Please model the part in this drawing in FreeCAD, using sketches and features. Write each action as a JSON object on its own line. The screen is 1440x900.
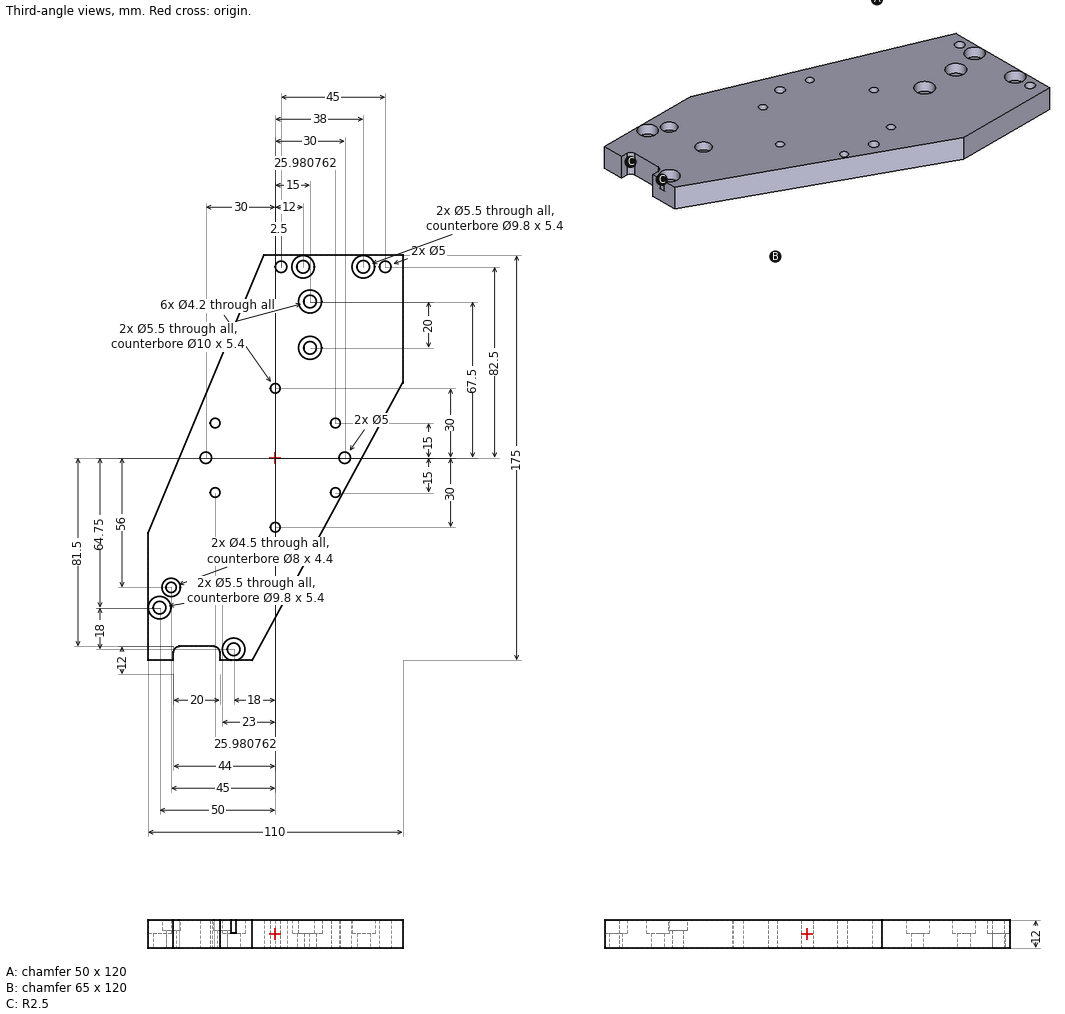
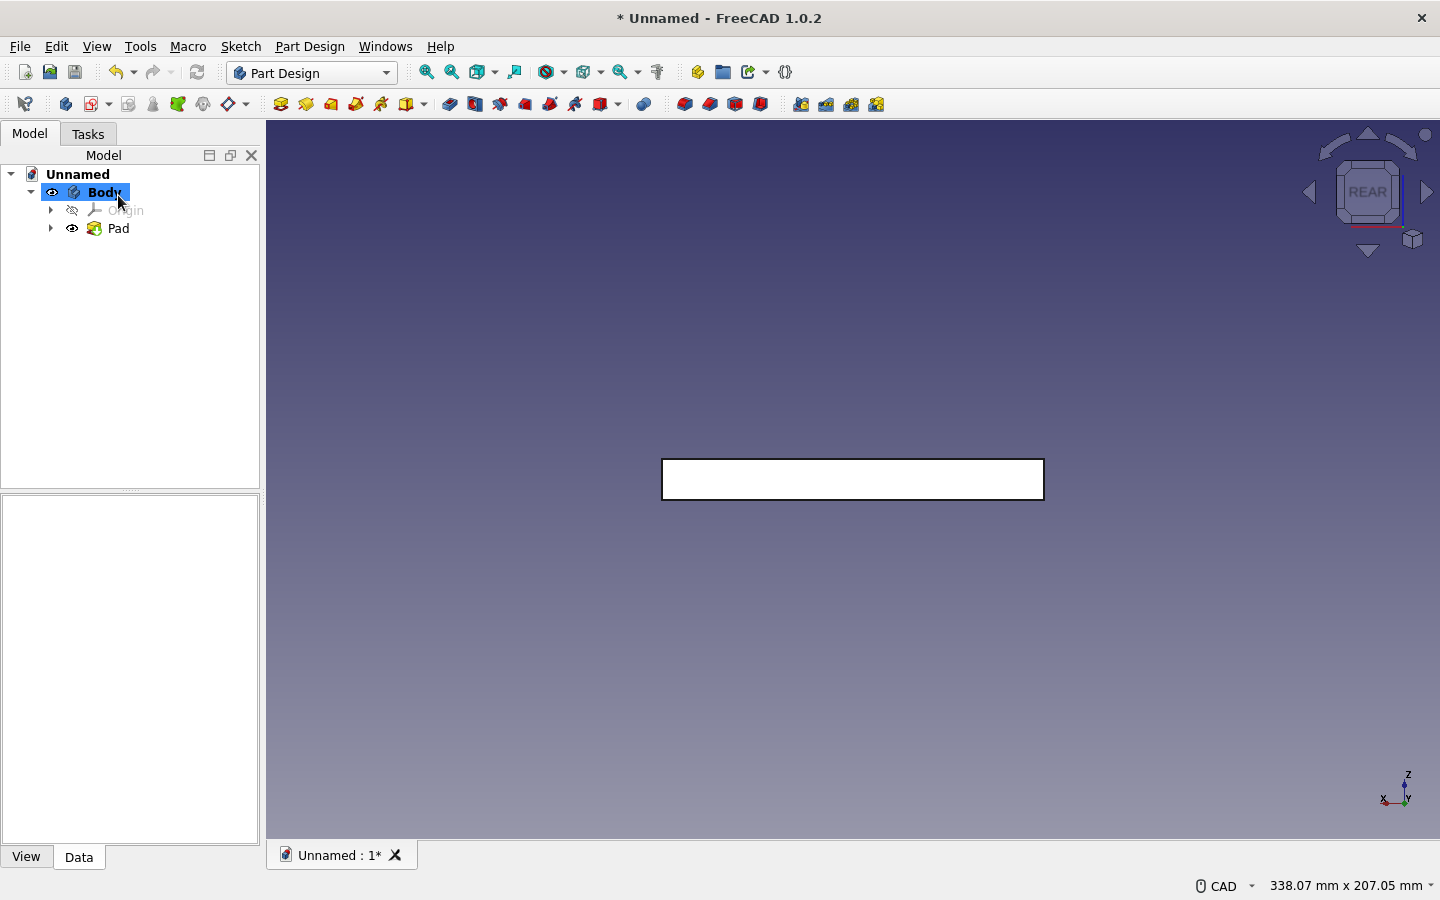
{"action": "left_click", "coordinate": [1044, 479]}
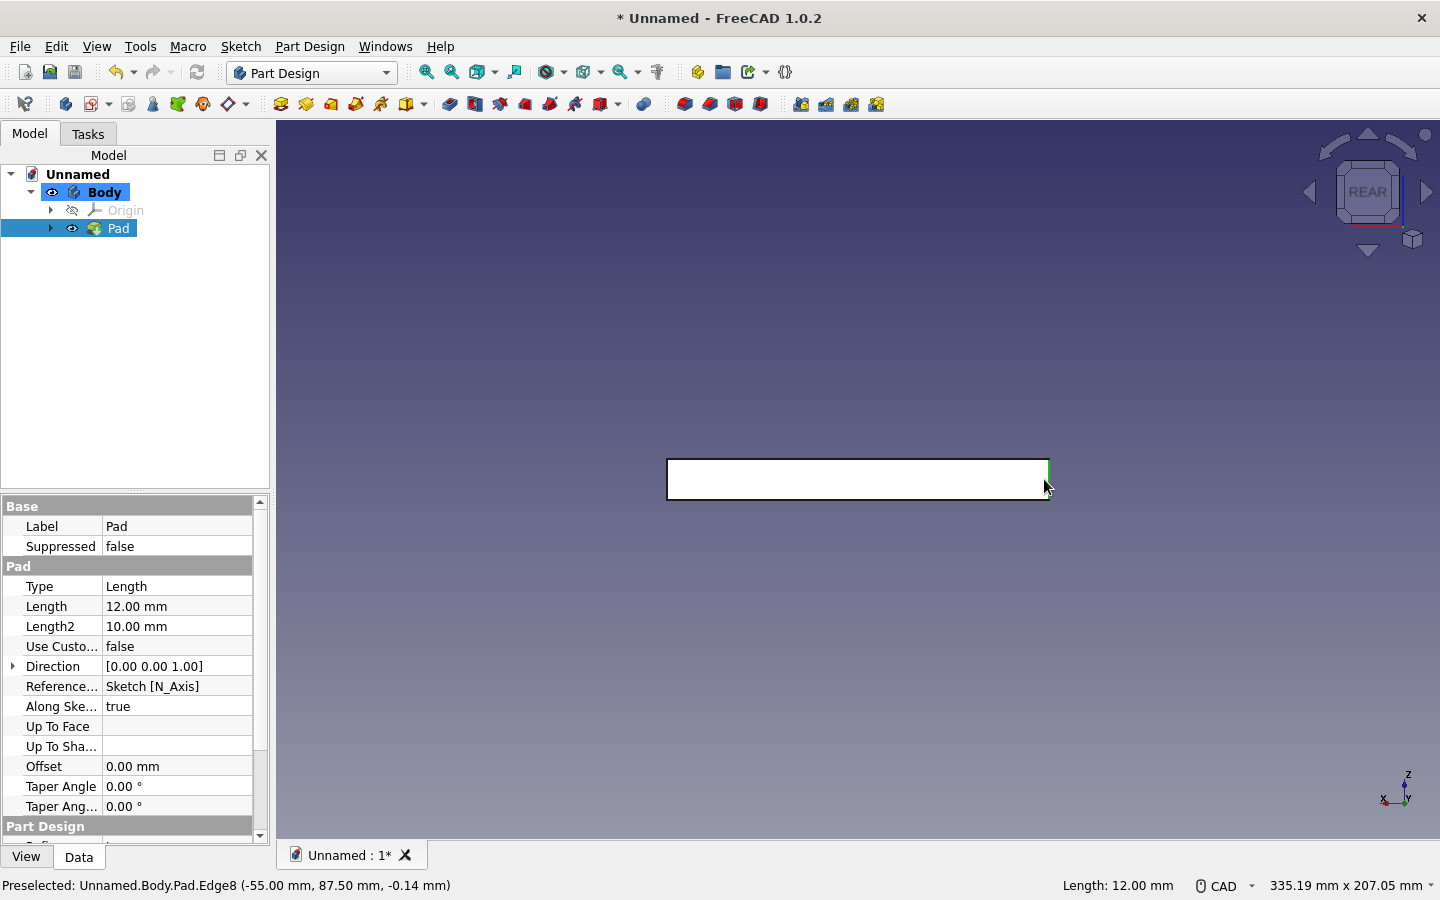
{"action": "left_click", "coordinate": [710, 104]}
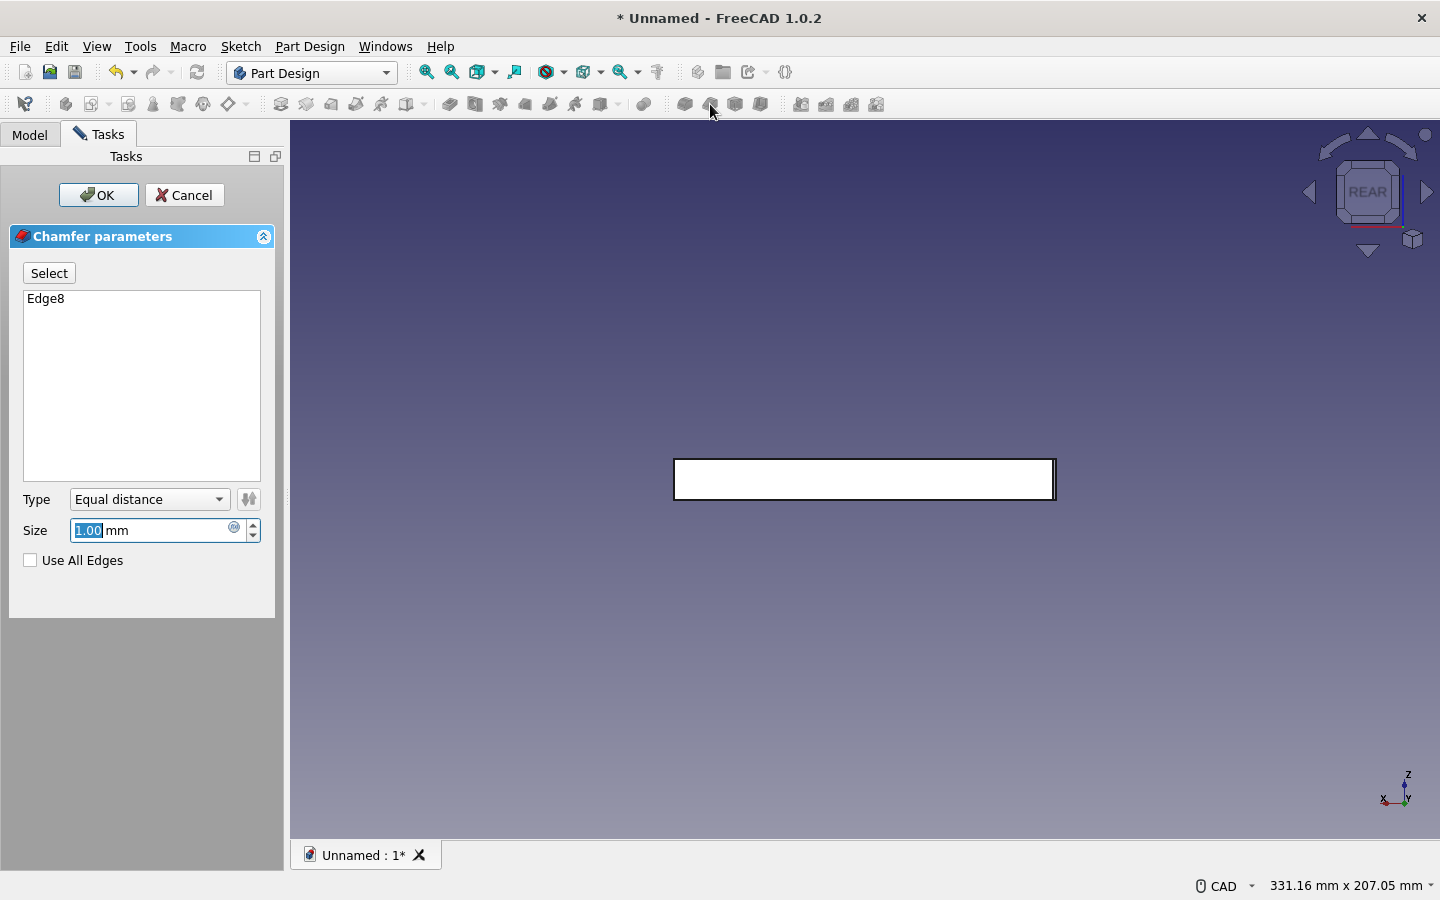
{"action": "type", "text": "50"}
{"action": "key", "text": "Tab"}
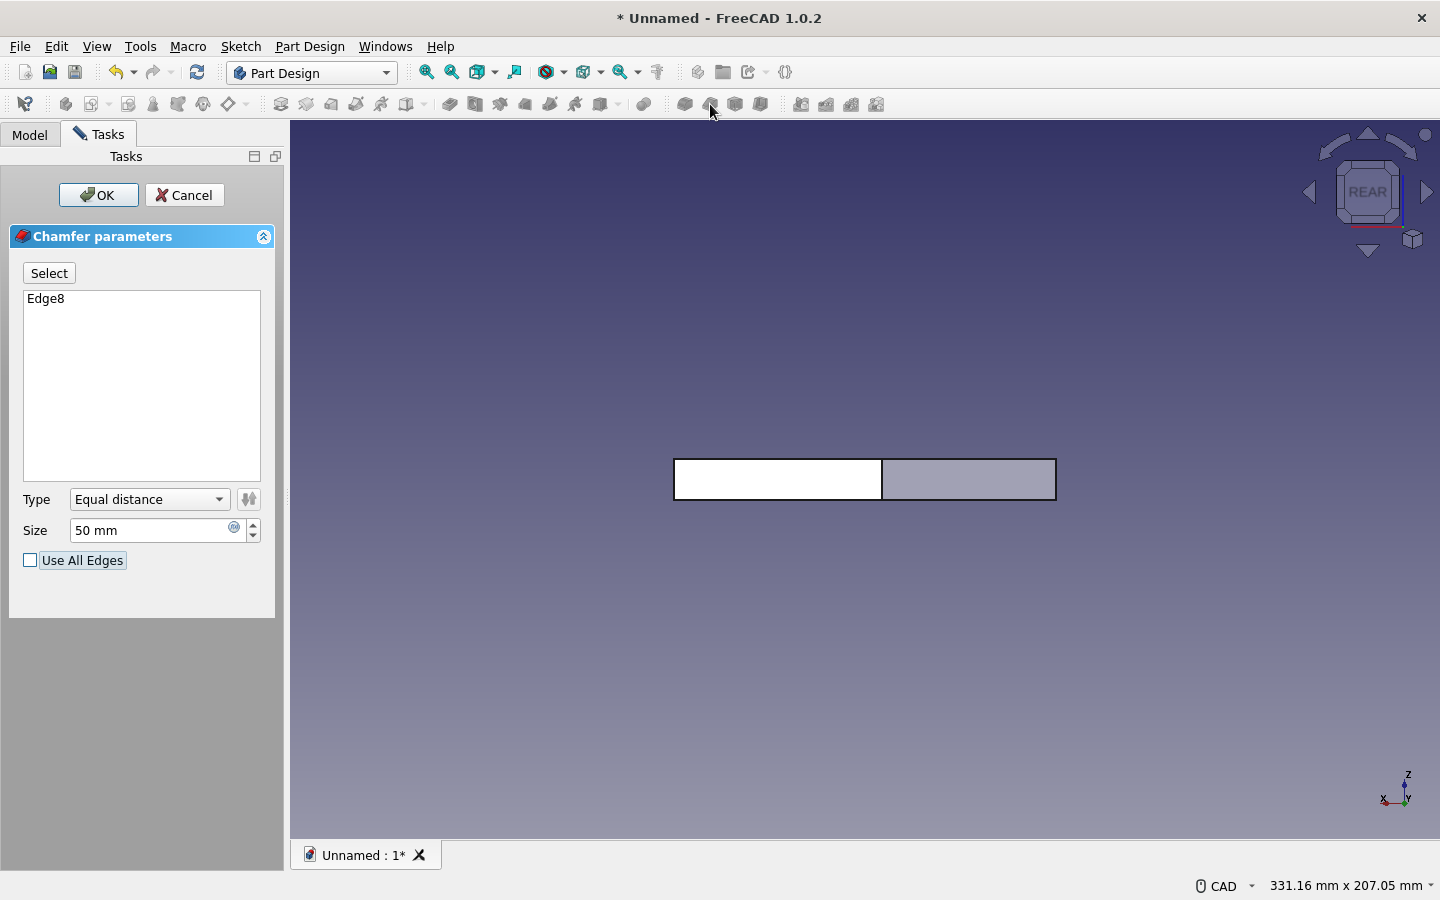
{"action": "left_click", "coordinate": [150, 500]}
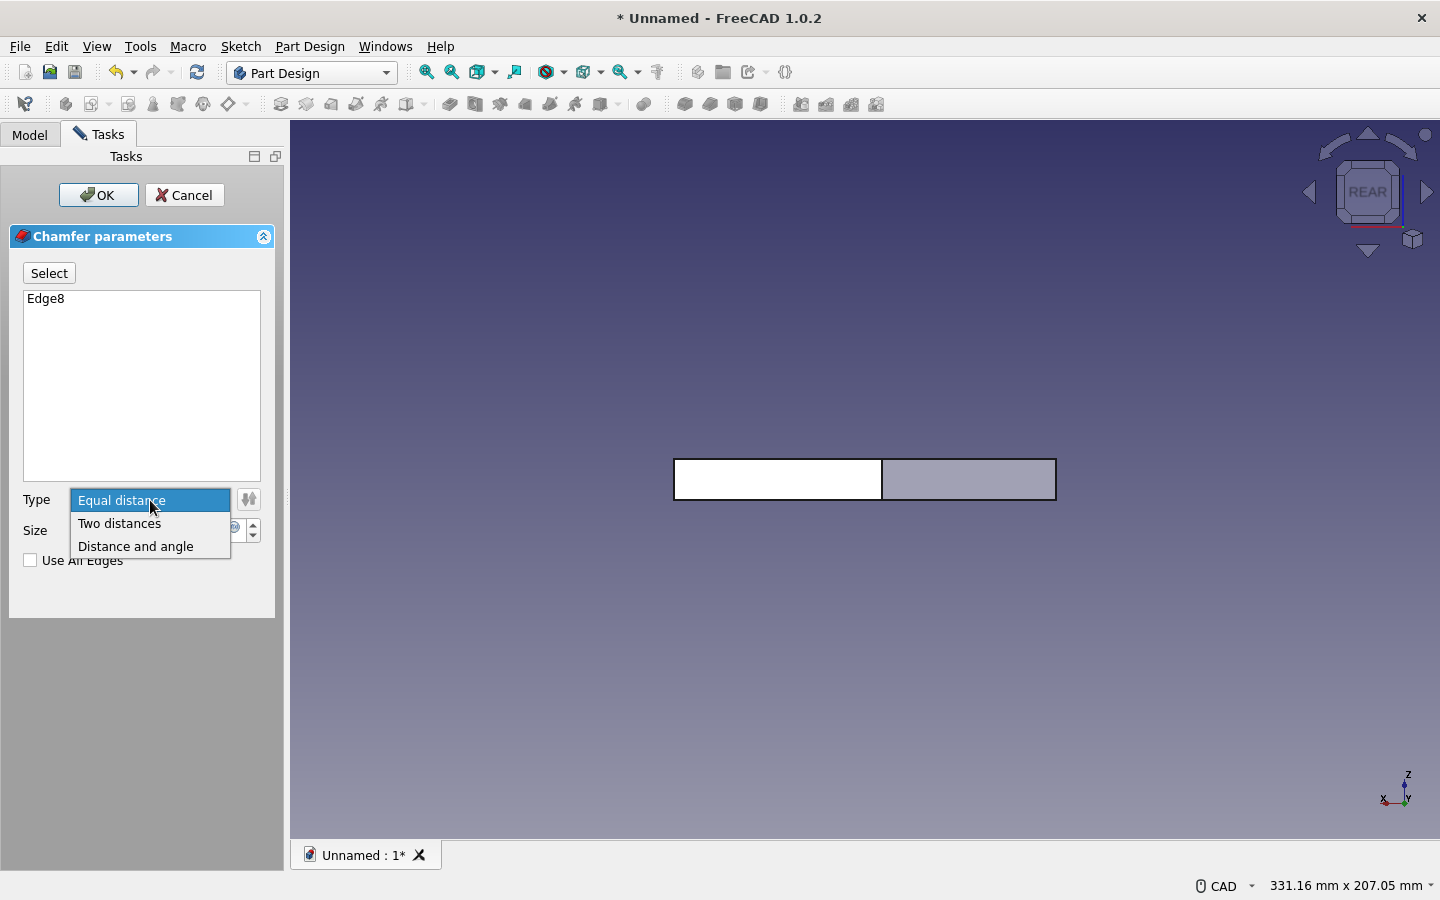
{"action": "left_click", "coordinate": [148, 524]}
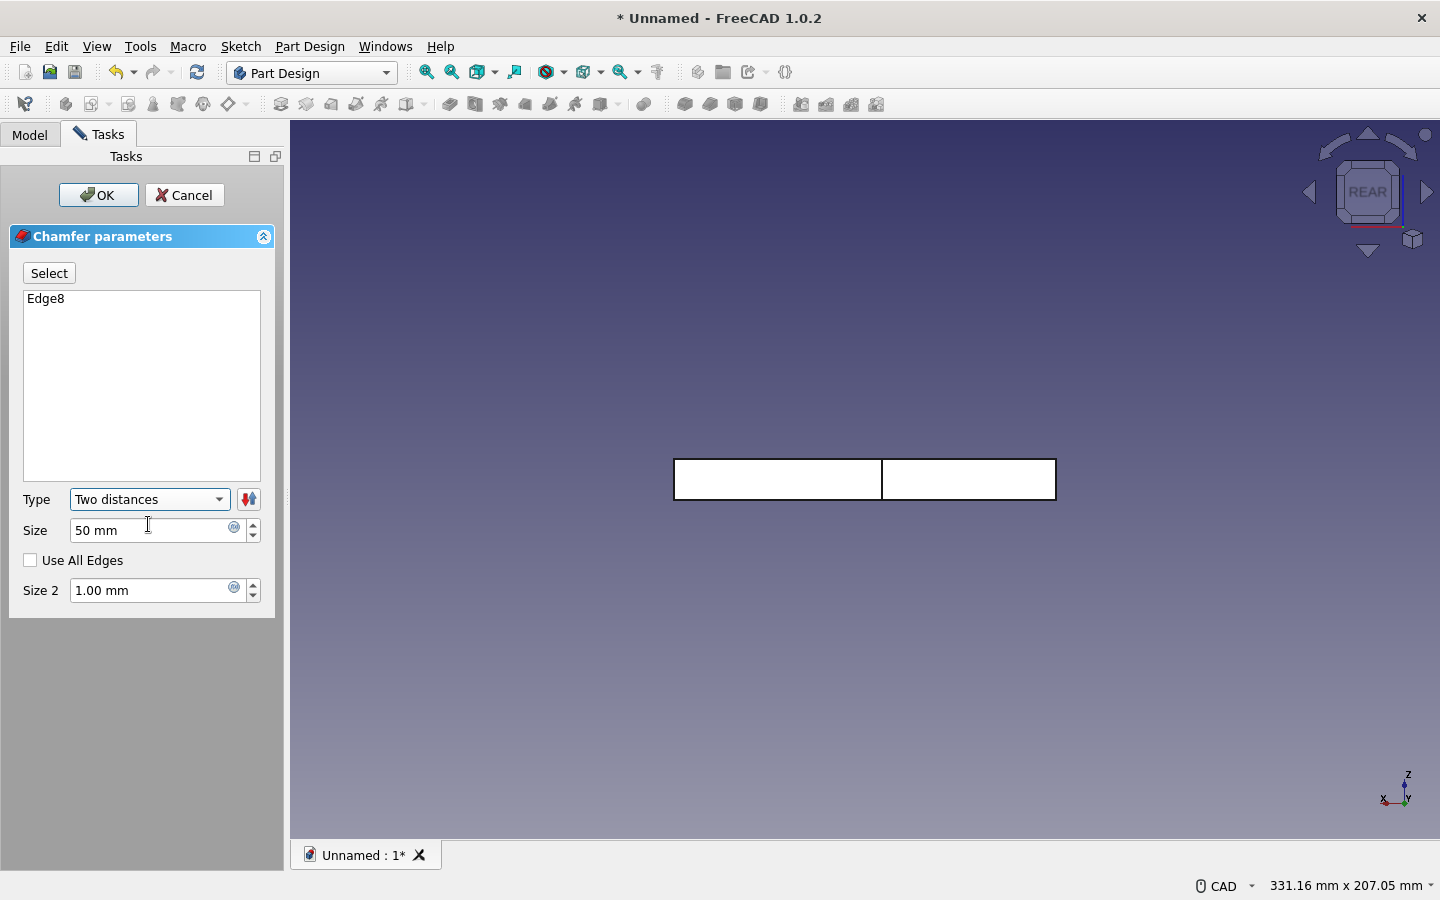
{"action": "triple_click", "coordinate": [158, 590]}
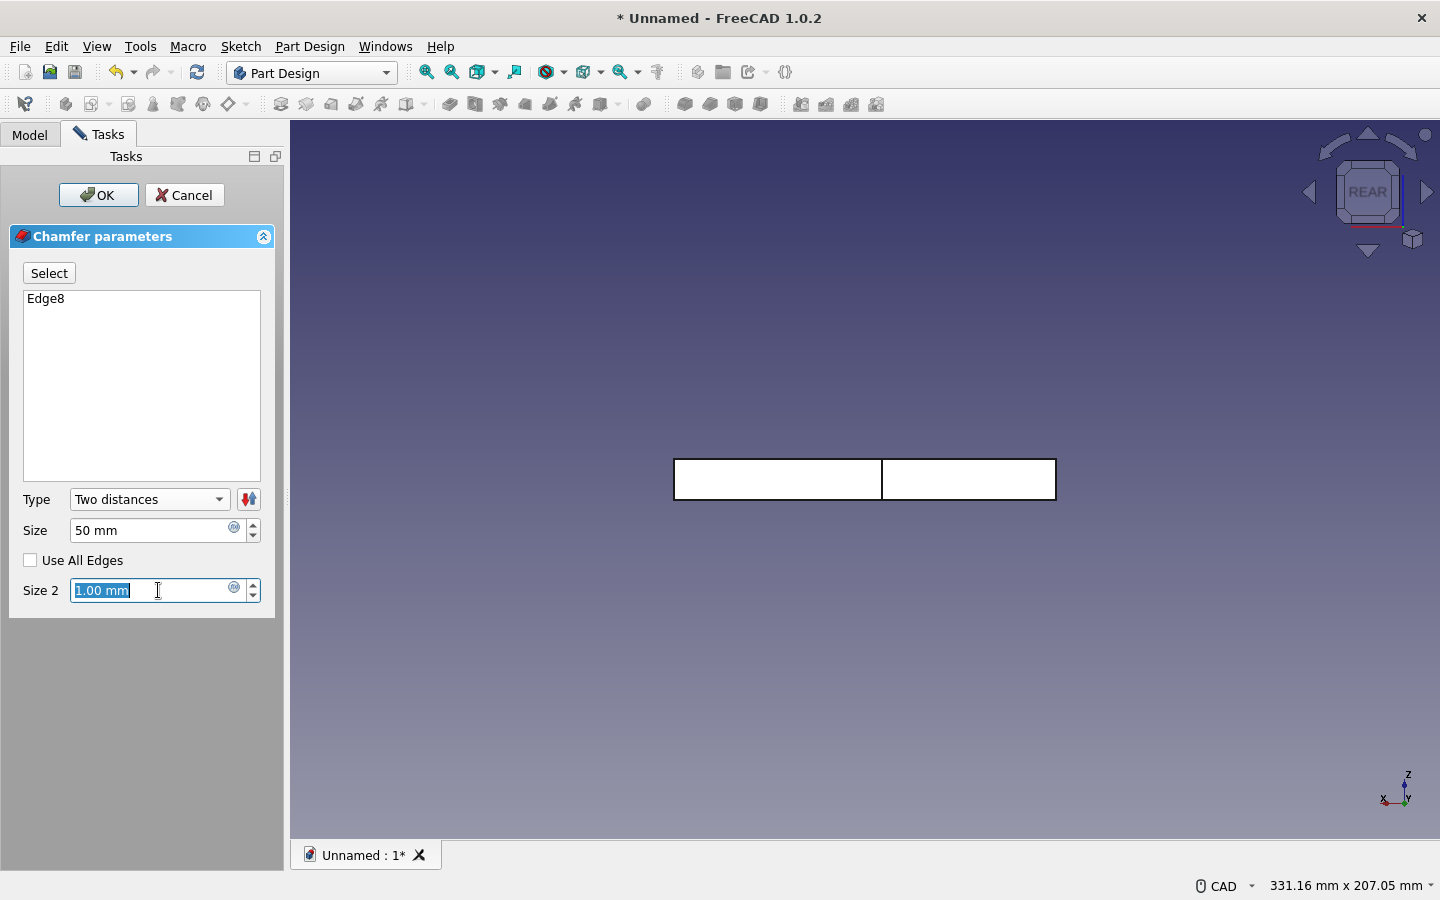
{"action": "type", "text": "120"}
{"action": "key", "text": "Tab"}